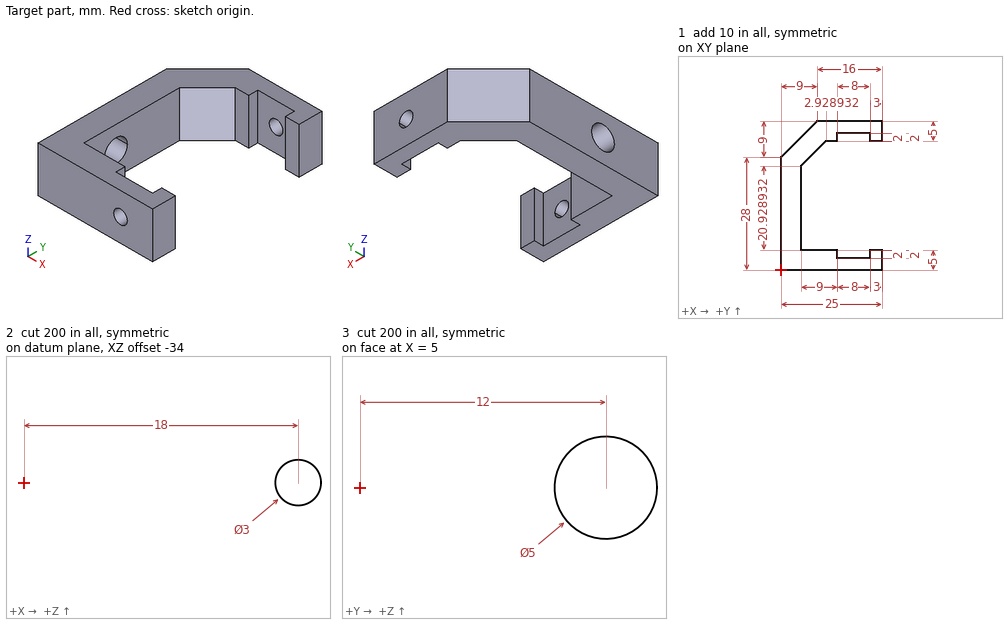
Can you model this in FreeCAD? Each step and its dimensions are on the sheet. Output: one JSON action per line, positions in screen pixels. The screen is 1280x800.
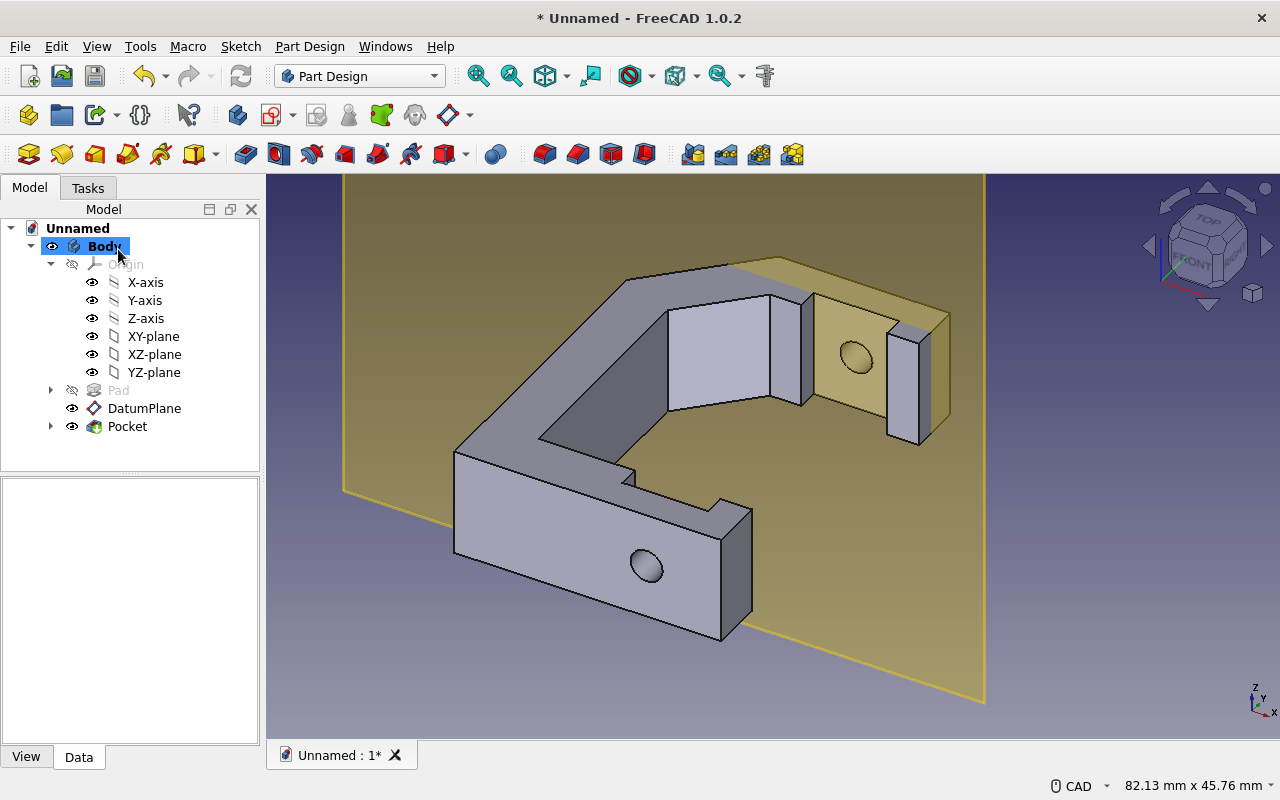
{"action": "left_click", "coordinate": [117, 408]}
{"action": "key", "text": "space"}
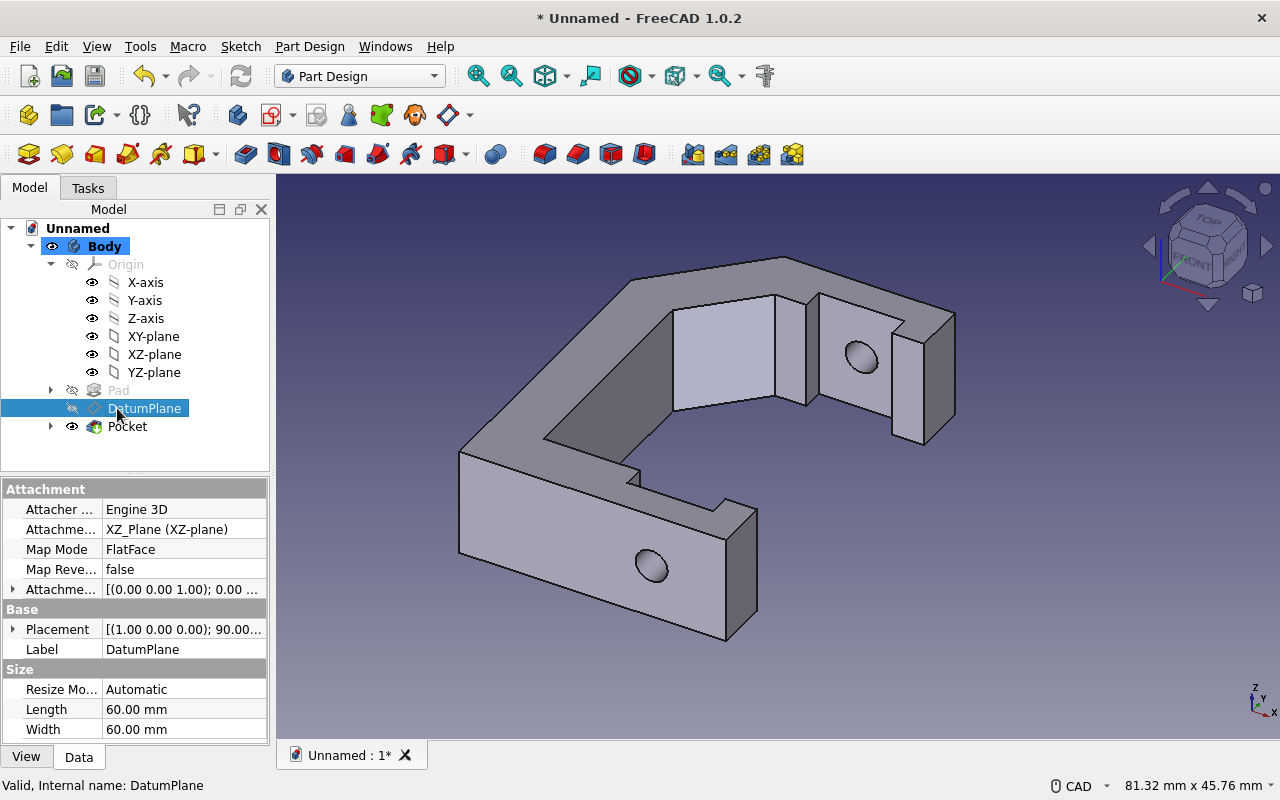
{"action": "left_click", "coordinate": [627, 406]}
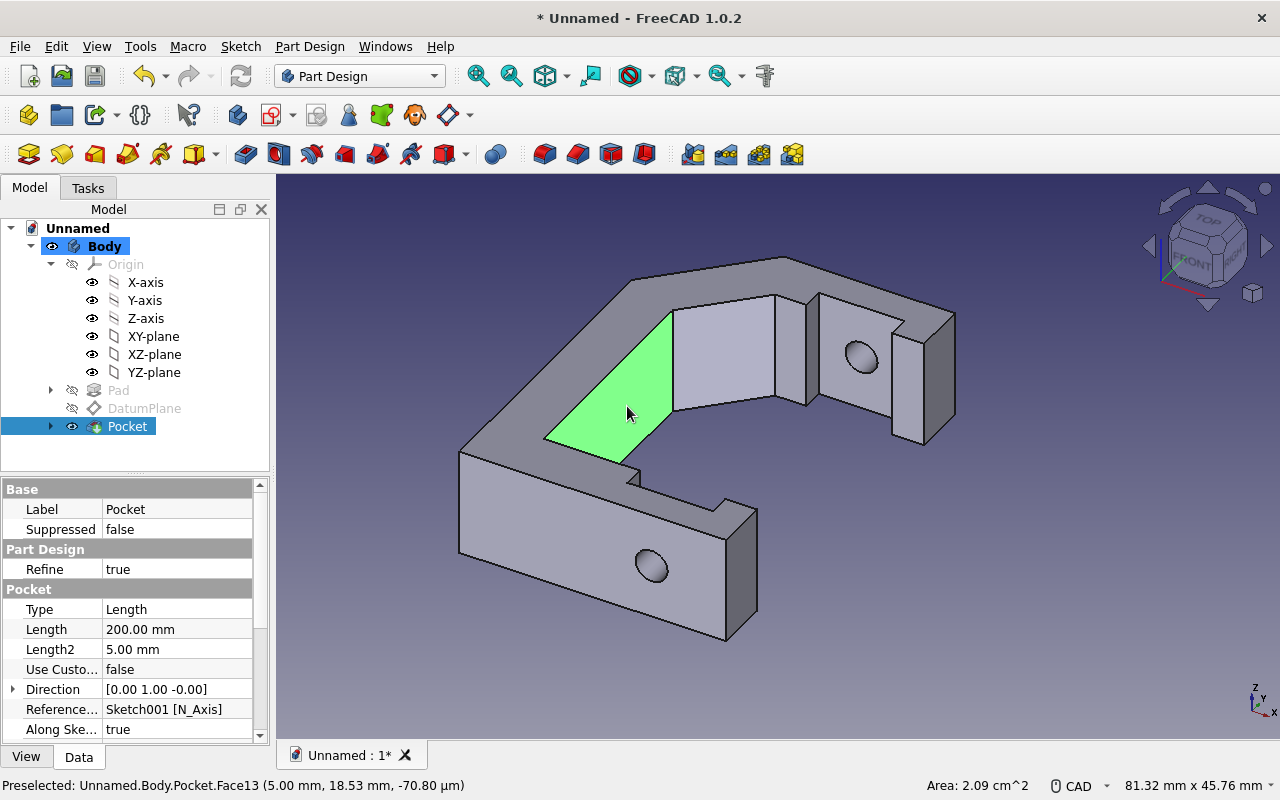
{"action": "left_click", "coordinate": [270, 116]}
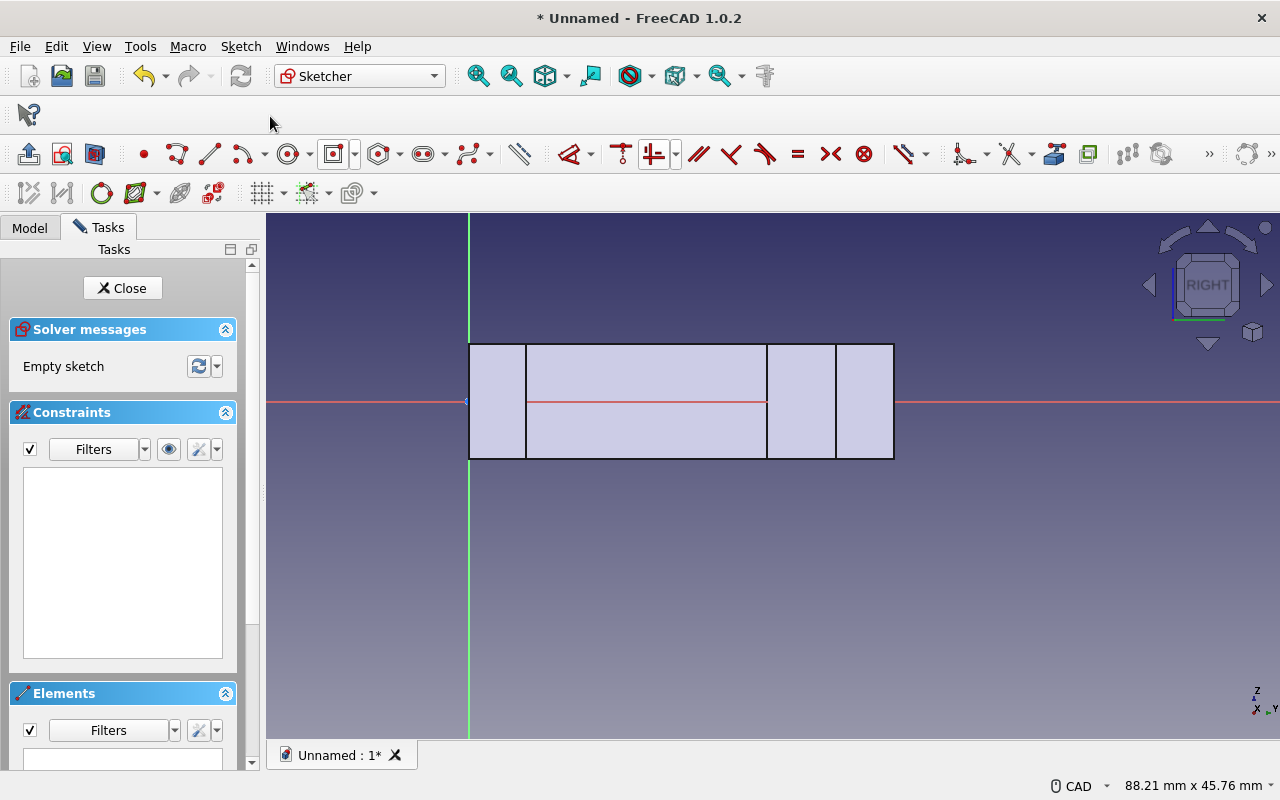
{"action": "scroll", "coordinate": [587, 387], "scroll_direction": "up", "scroll_amount": 9}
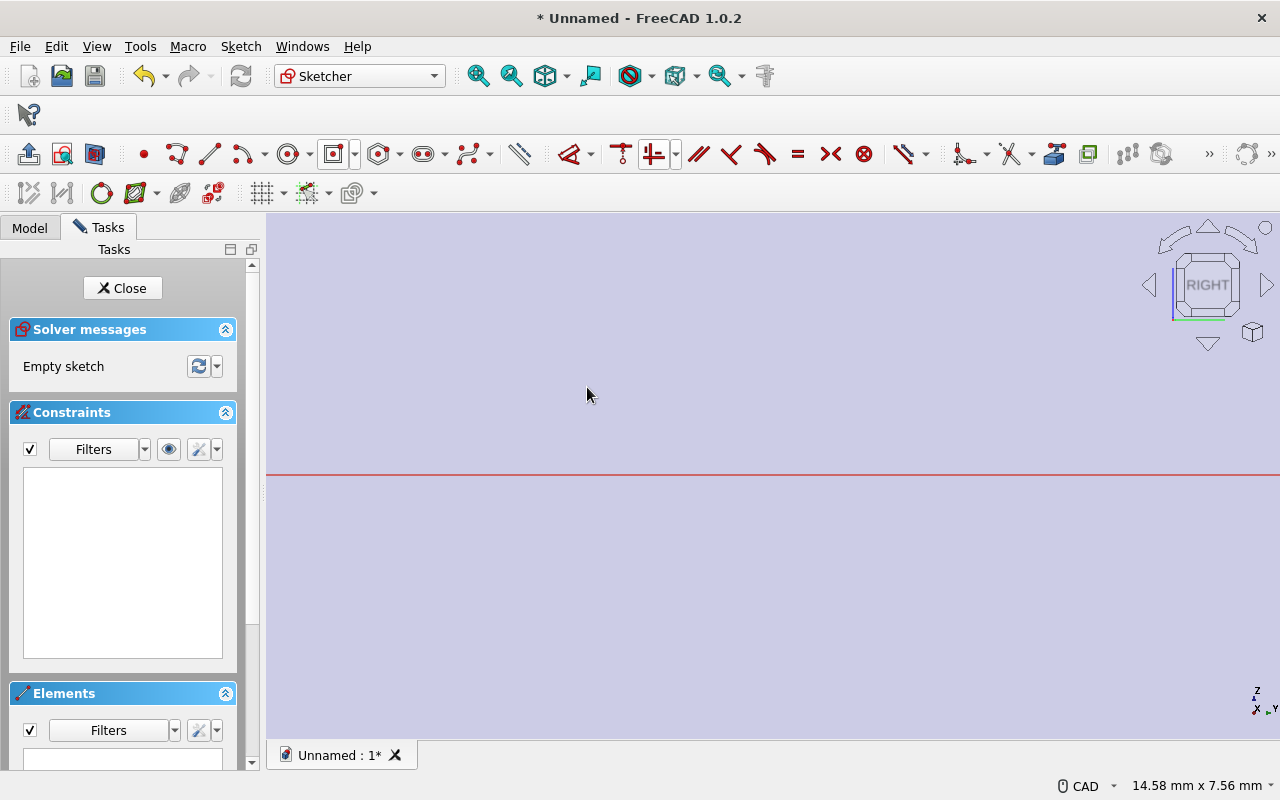
{"action": "key", "text": "g c"}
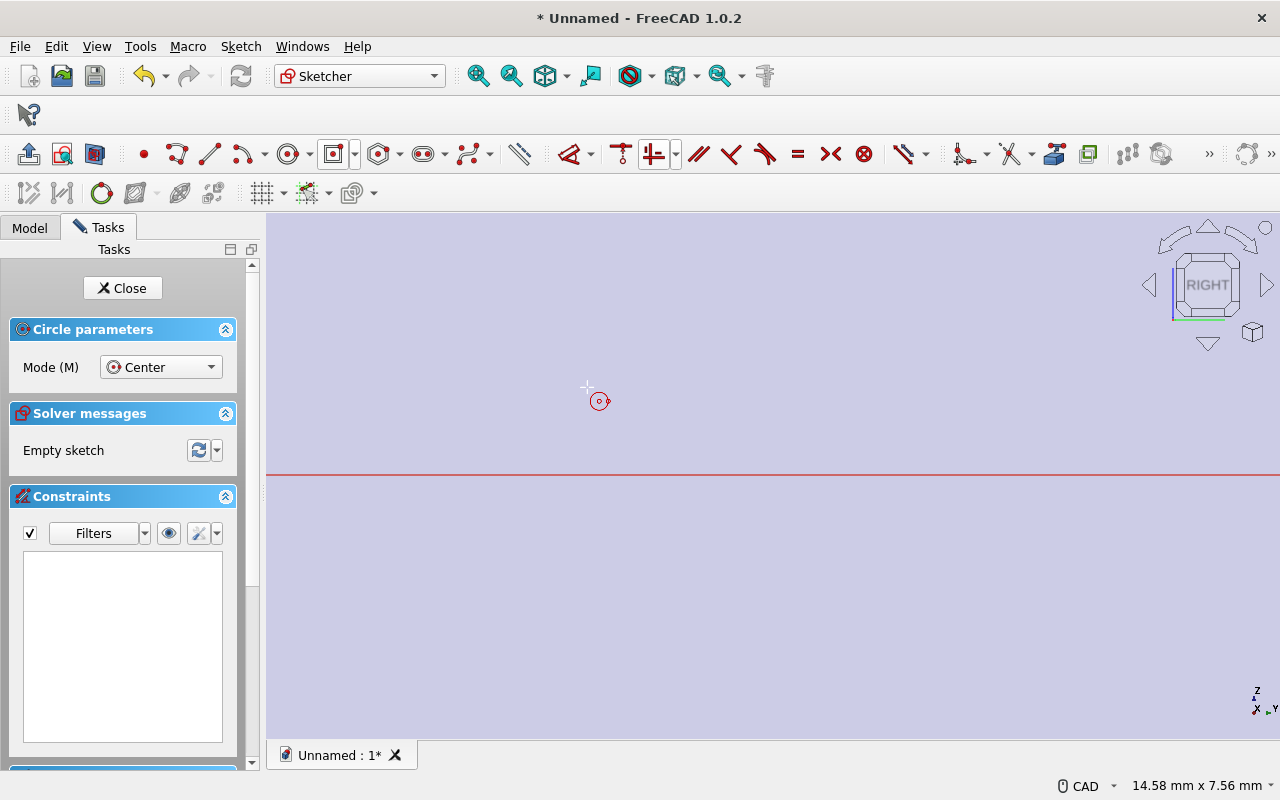
{"action": "left_click", "coordinate": [703, 475]}
{"action": "left_click", "coordinate": [826, 352]}
{"action": "key", "text": "Escape"}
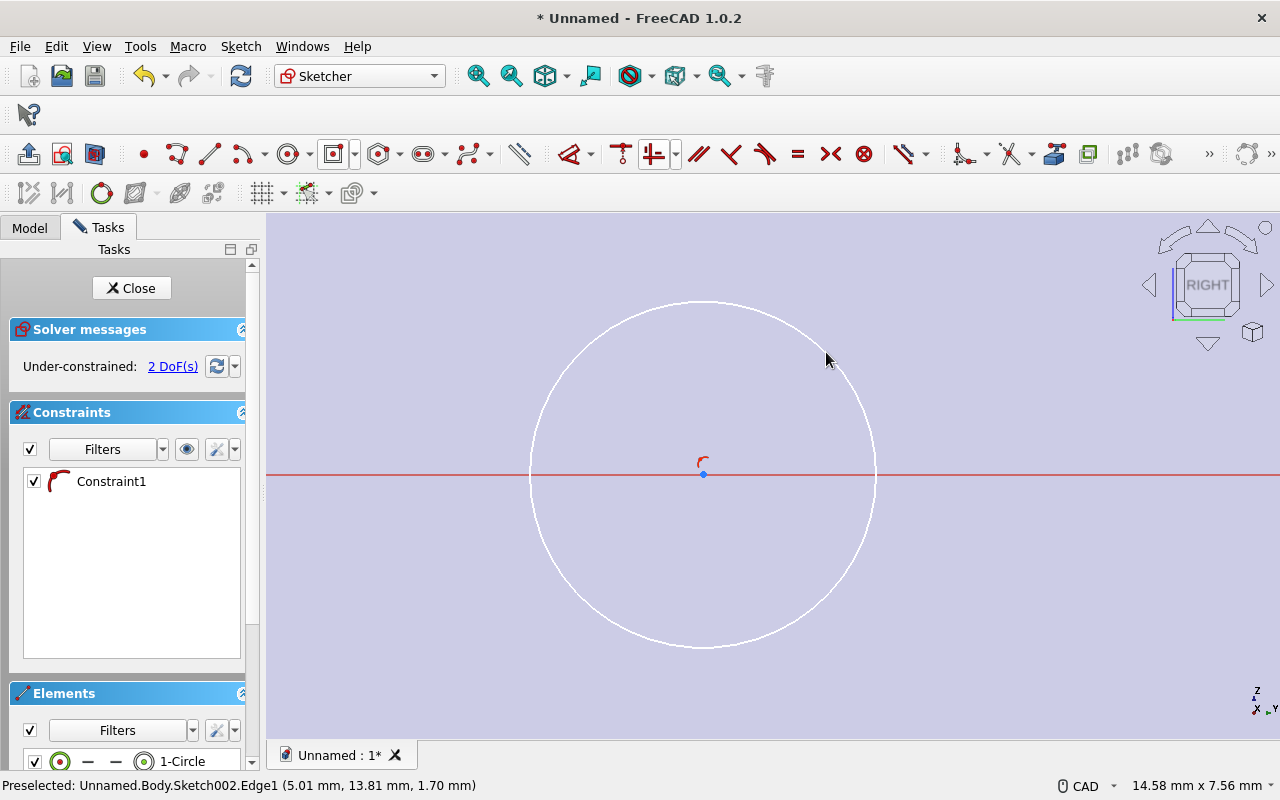
{"action": "key", "text": "d"}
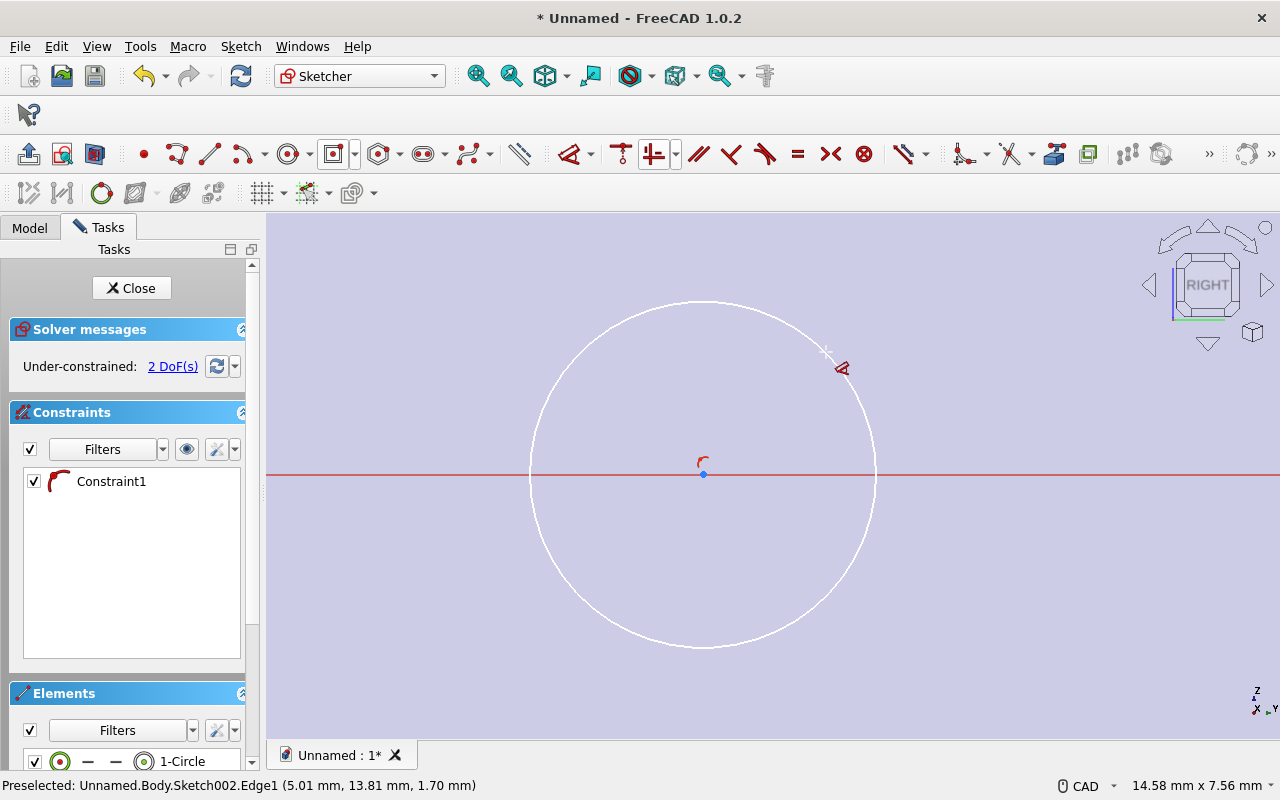
{"action": "left_click", "coordinate": [825, 352]}
{"action": "left_click", "coordinate": [848, 329]}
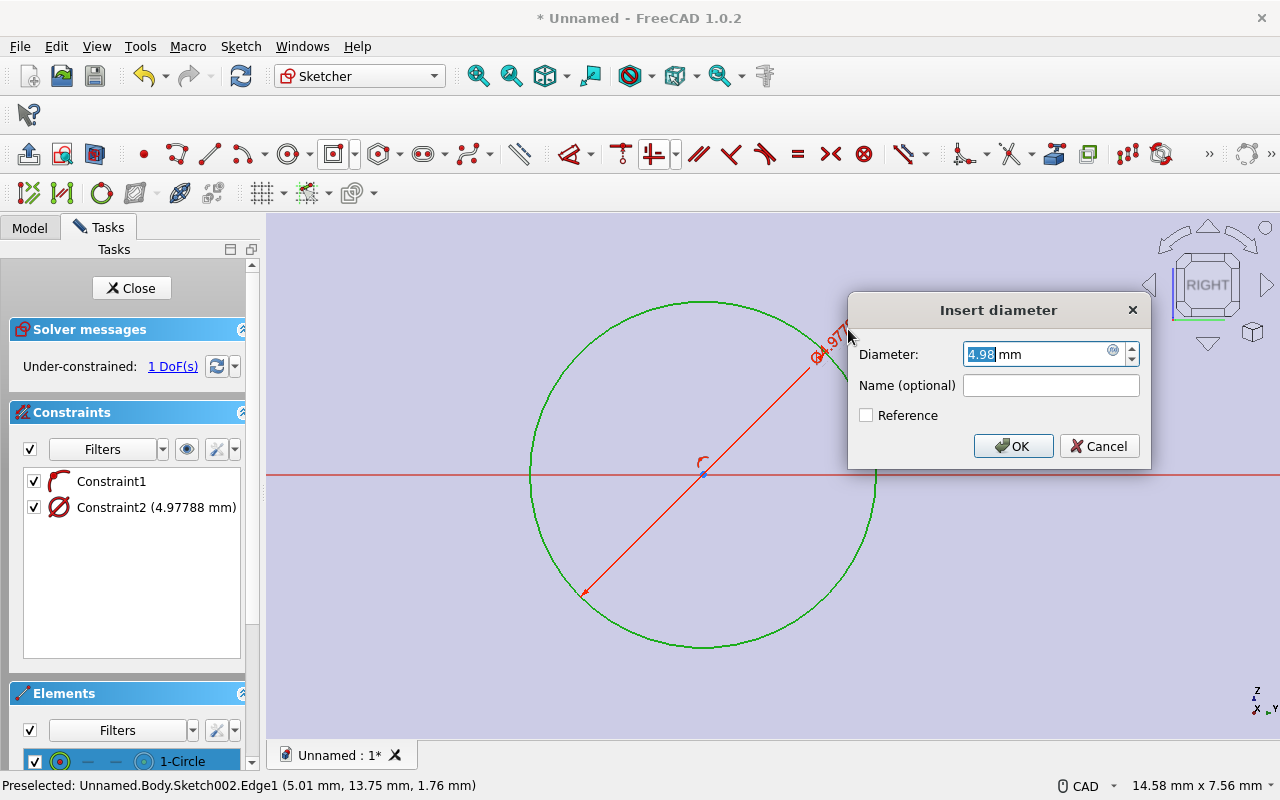
{"action": "type", "text": "5"}
{"action": "key", "text": "Return"}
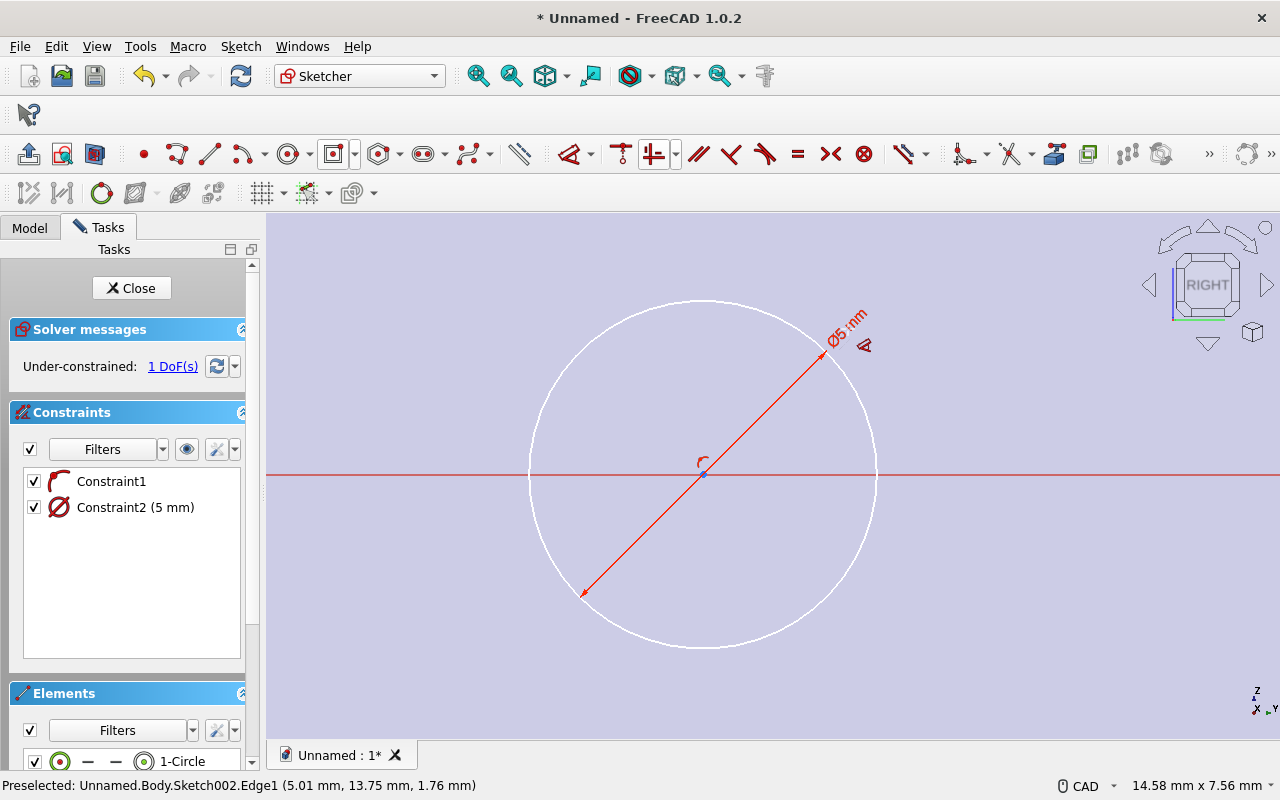
{"action": "left_click", "coordinate": [703, 475]}
{"action": "left_click", "coordinate": [498, 509]}